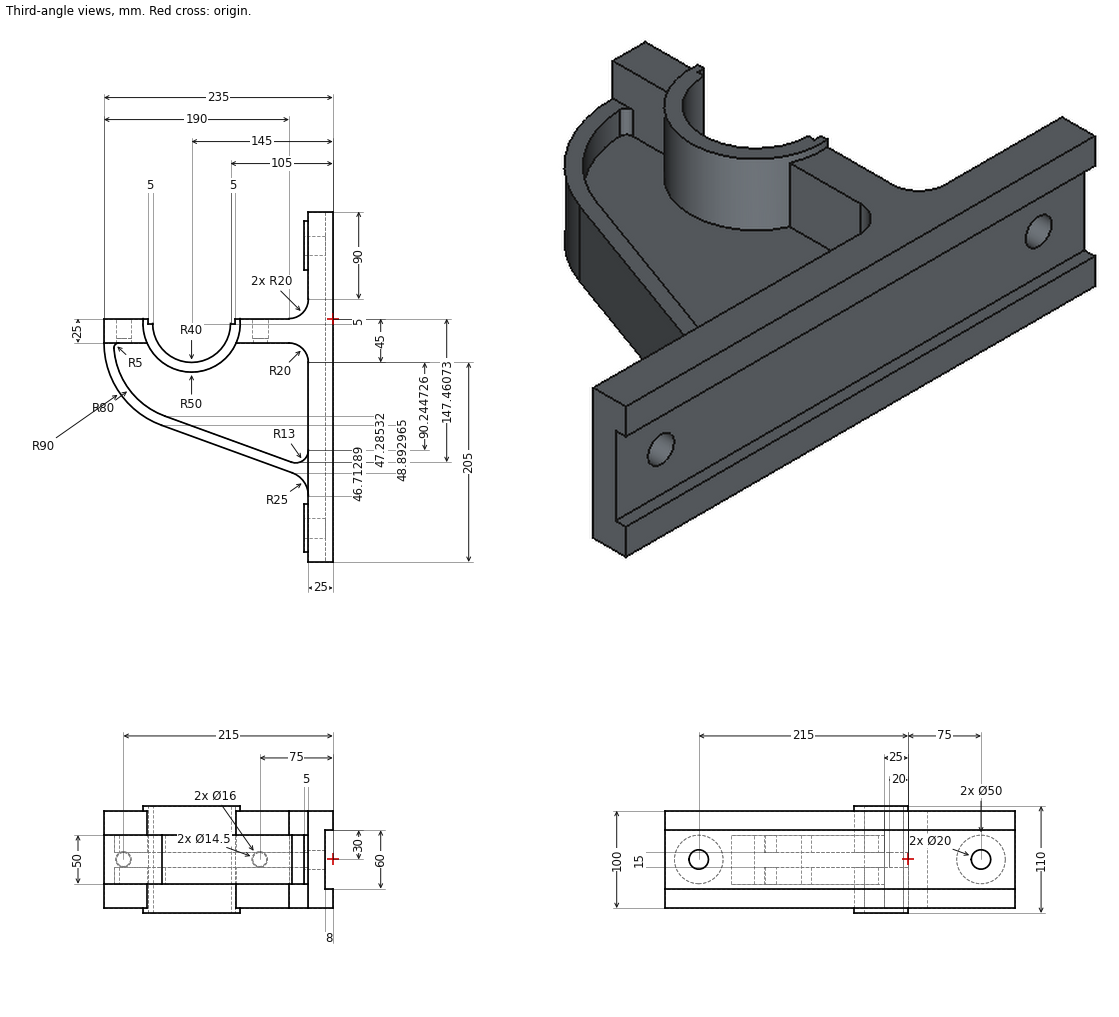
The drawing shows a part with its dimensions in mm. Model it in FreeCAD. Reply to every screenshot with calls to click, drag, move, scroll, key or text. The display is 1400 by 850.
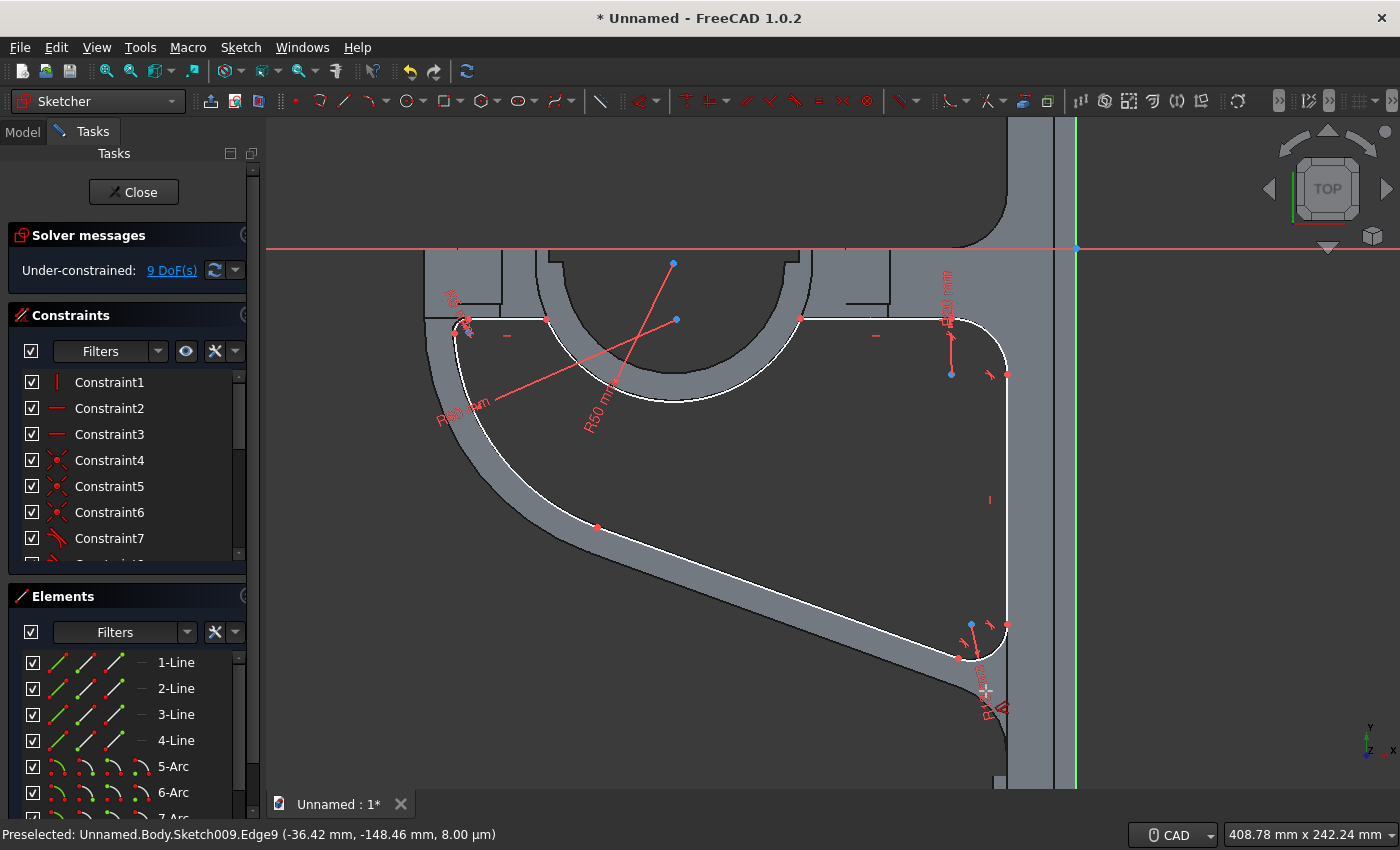
scroll(674, 263, up, 6)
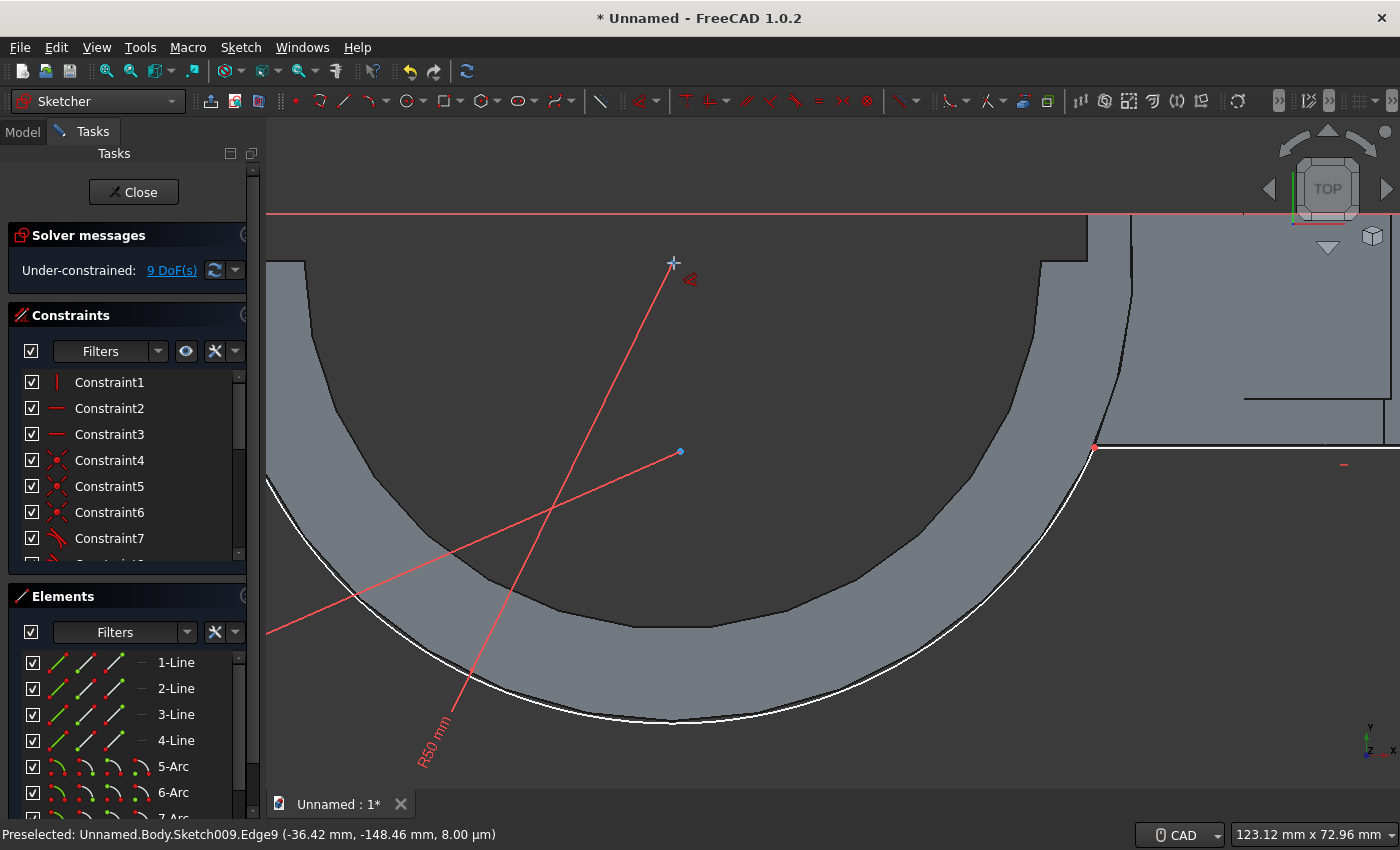
click(673, 263)
click(639, 239)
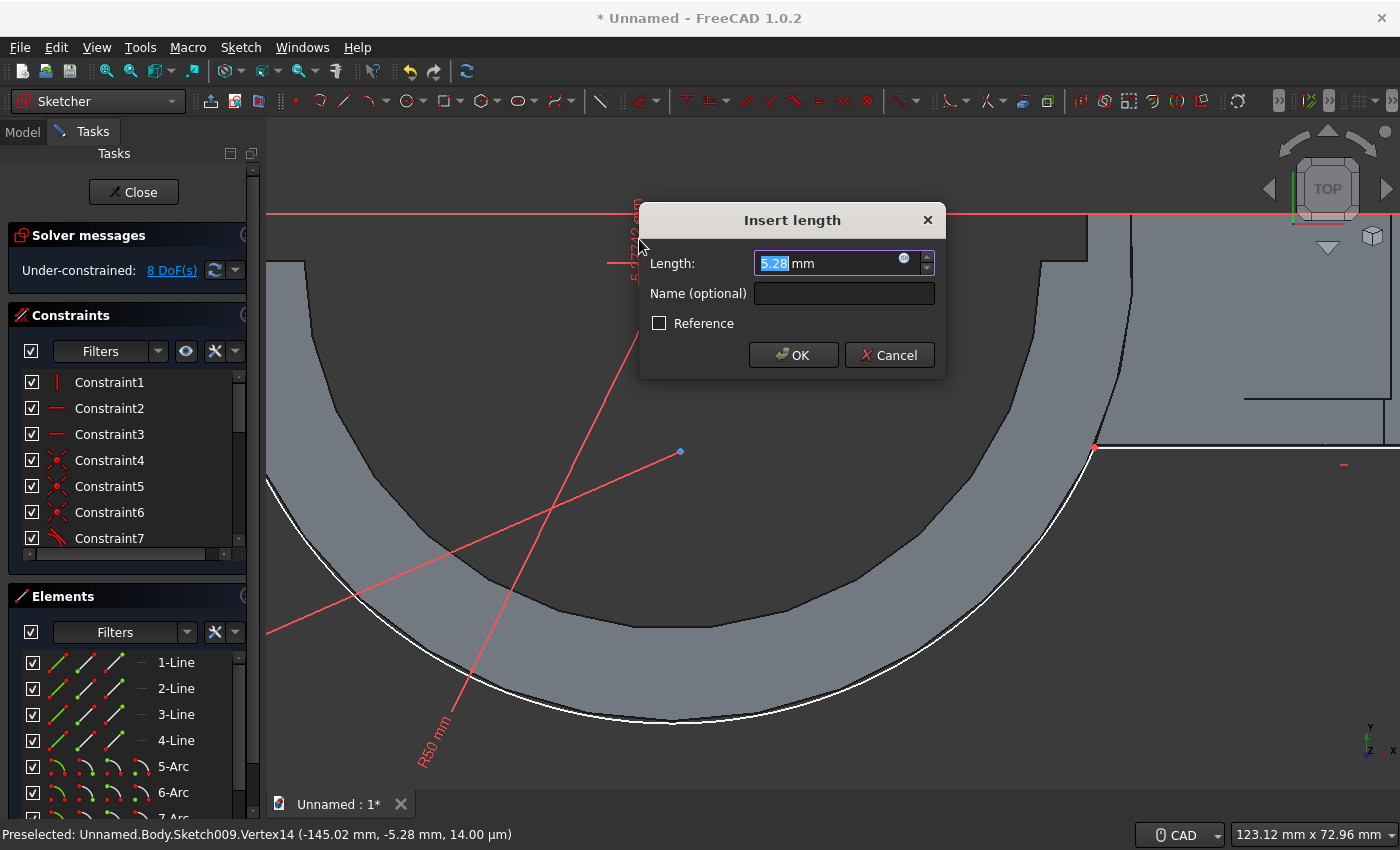
text(5)
key(Return)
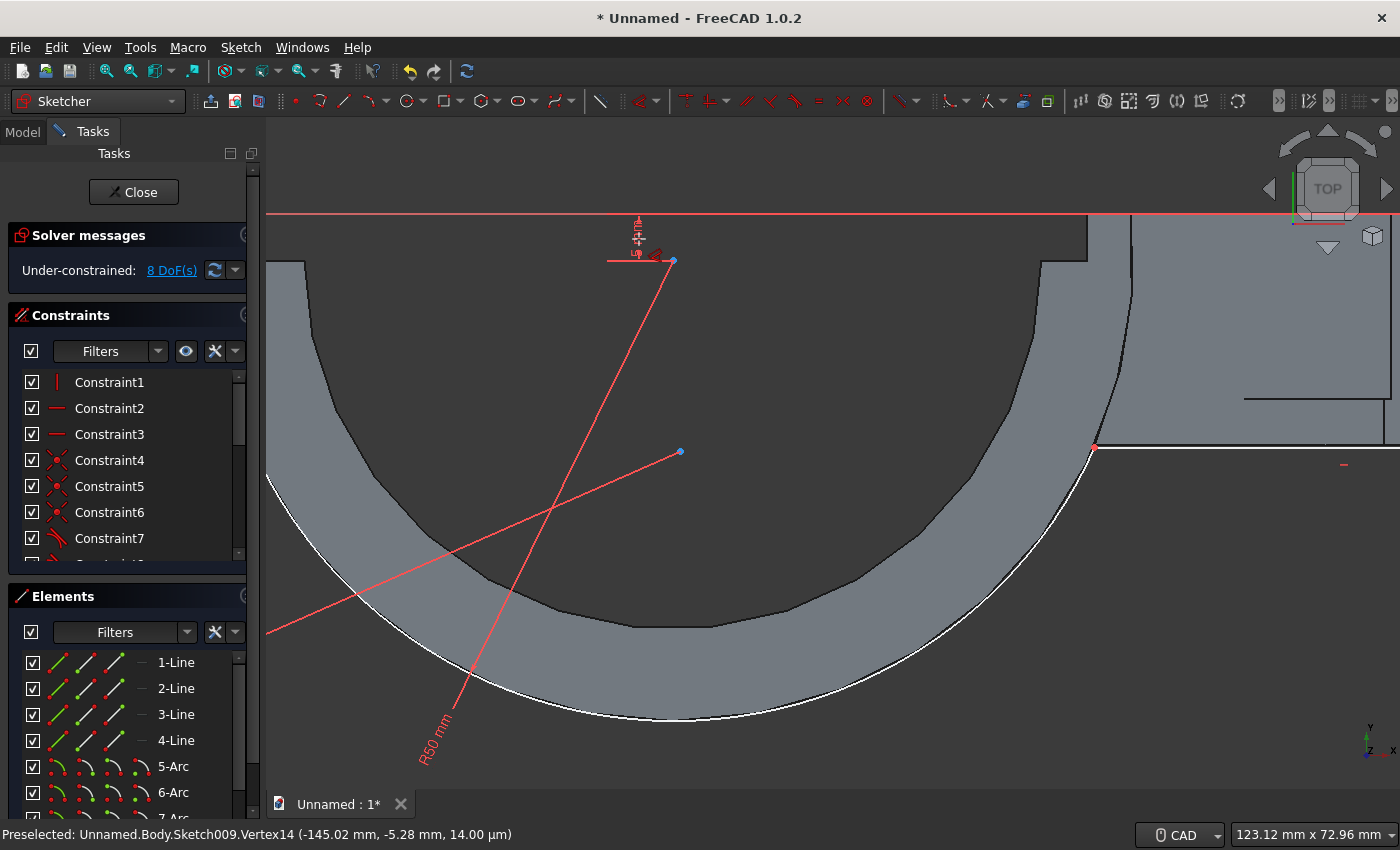
scroll(675, 263, down, 6)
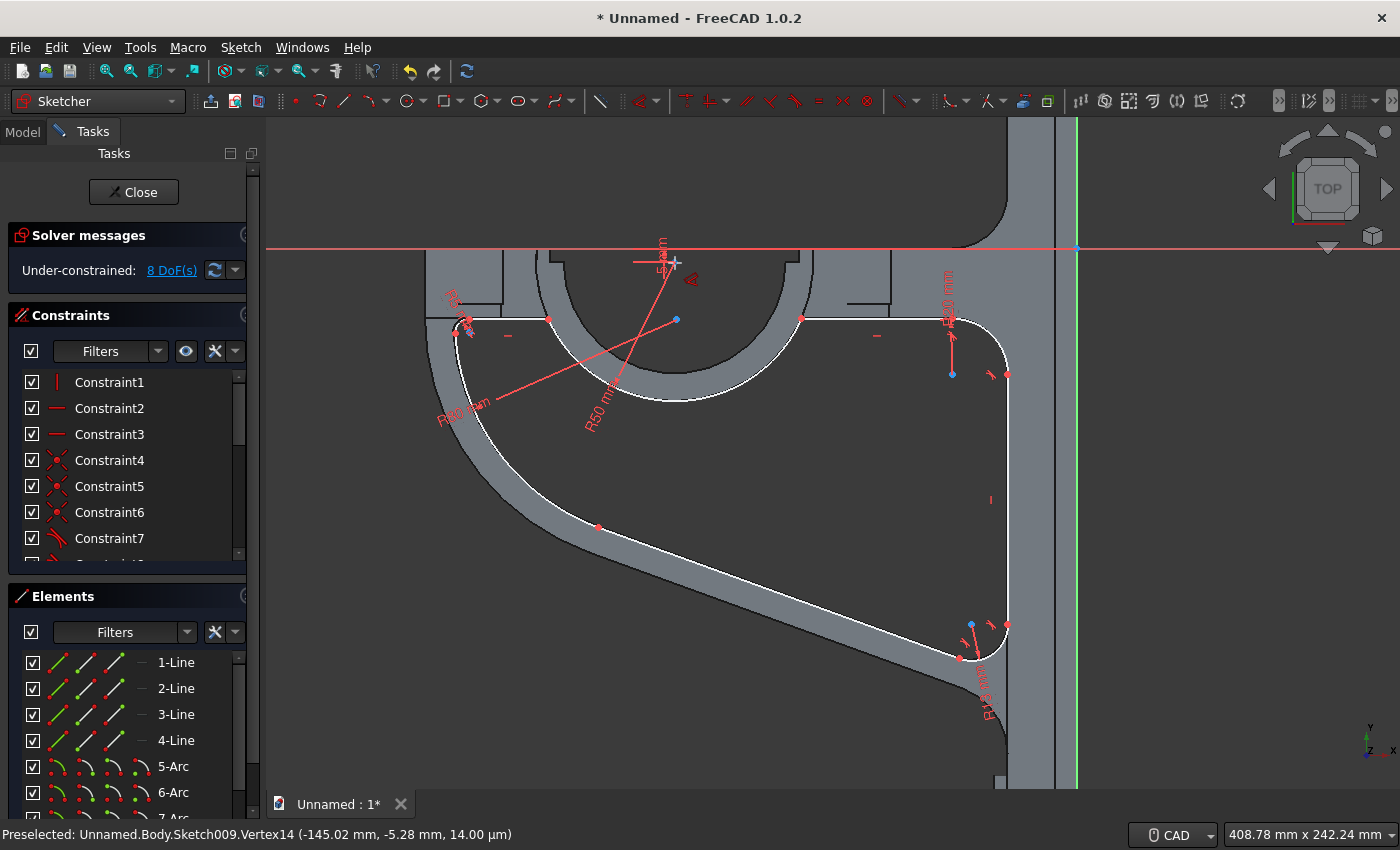
click(1008, 625)
click(1042, 215)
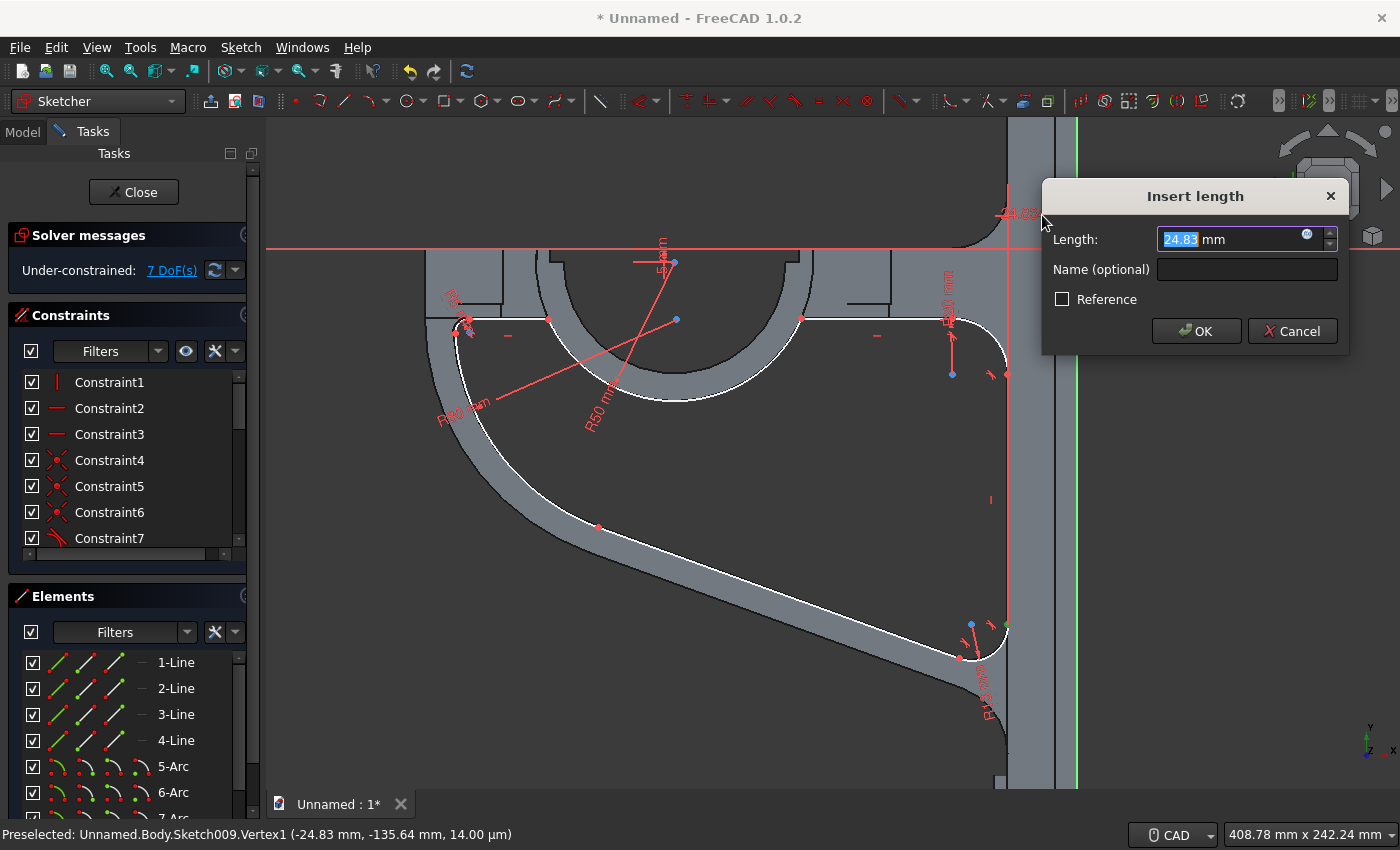
text(25)
key(Return)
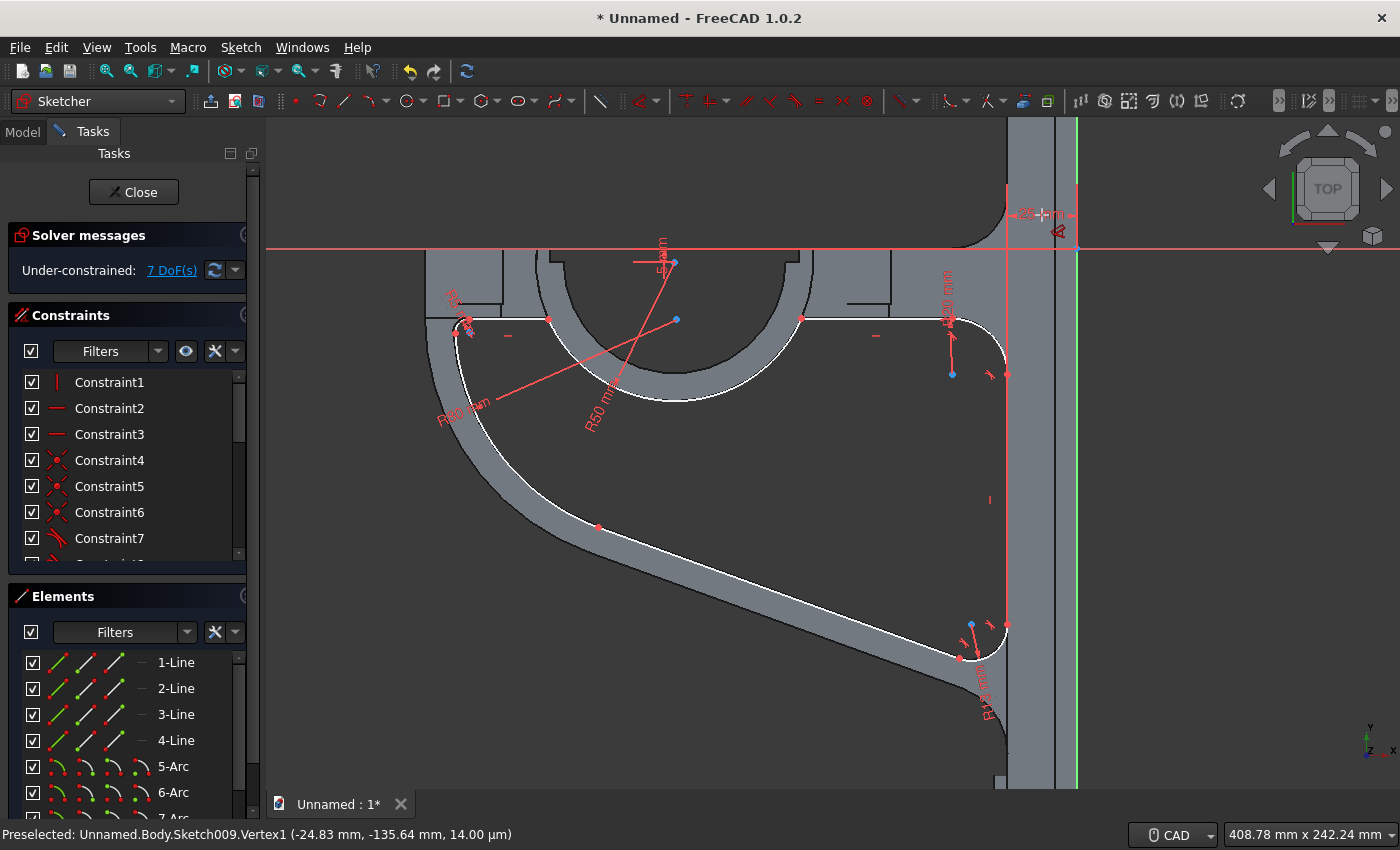
click(1007, 374)
click(1111, 311)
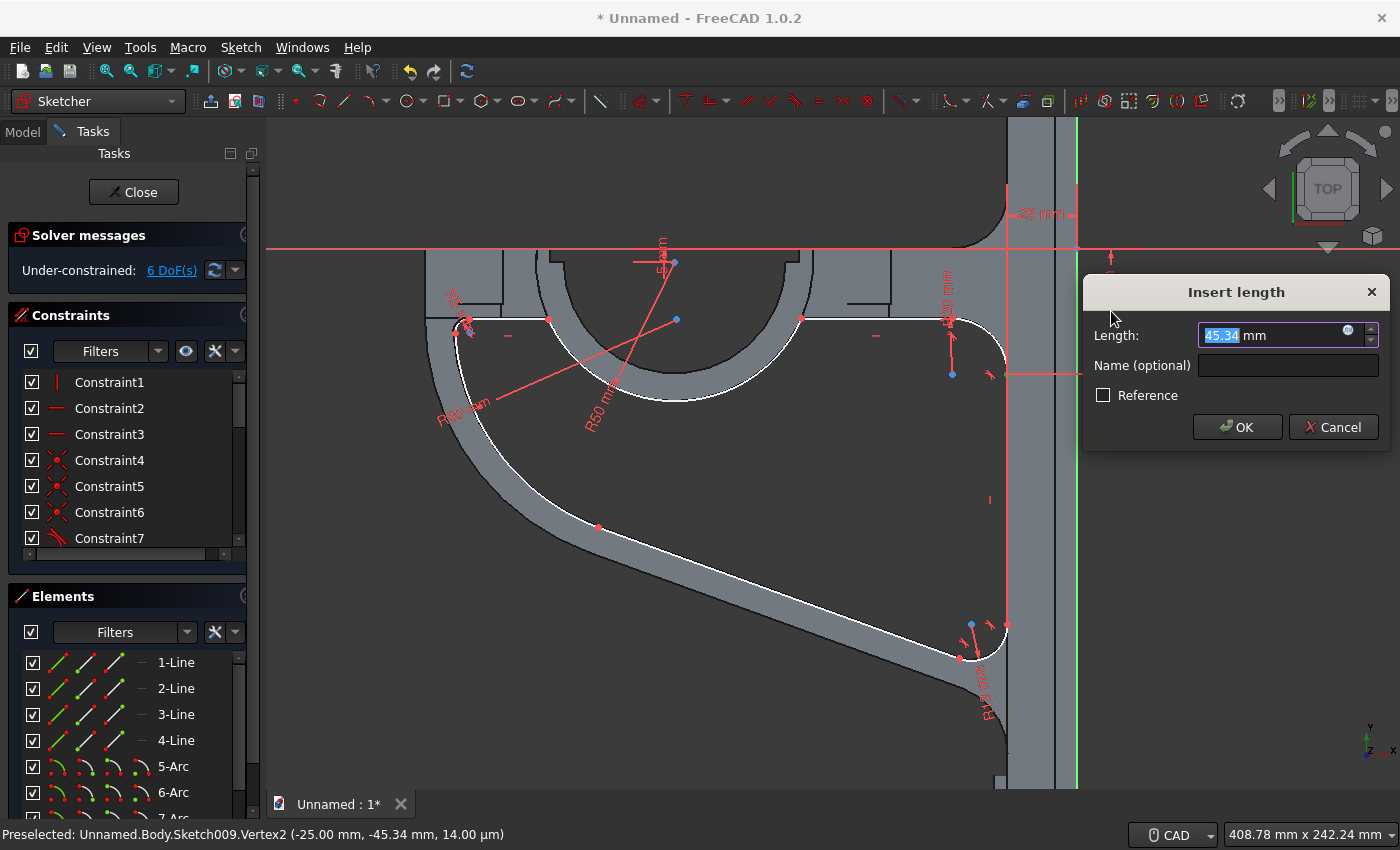
text(45)
key(Return)